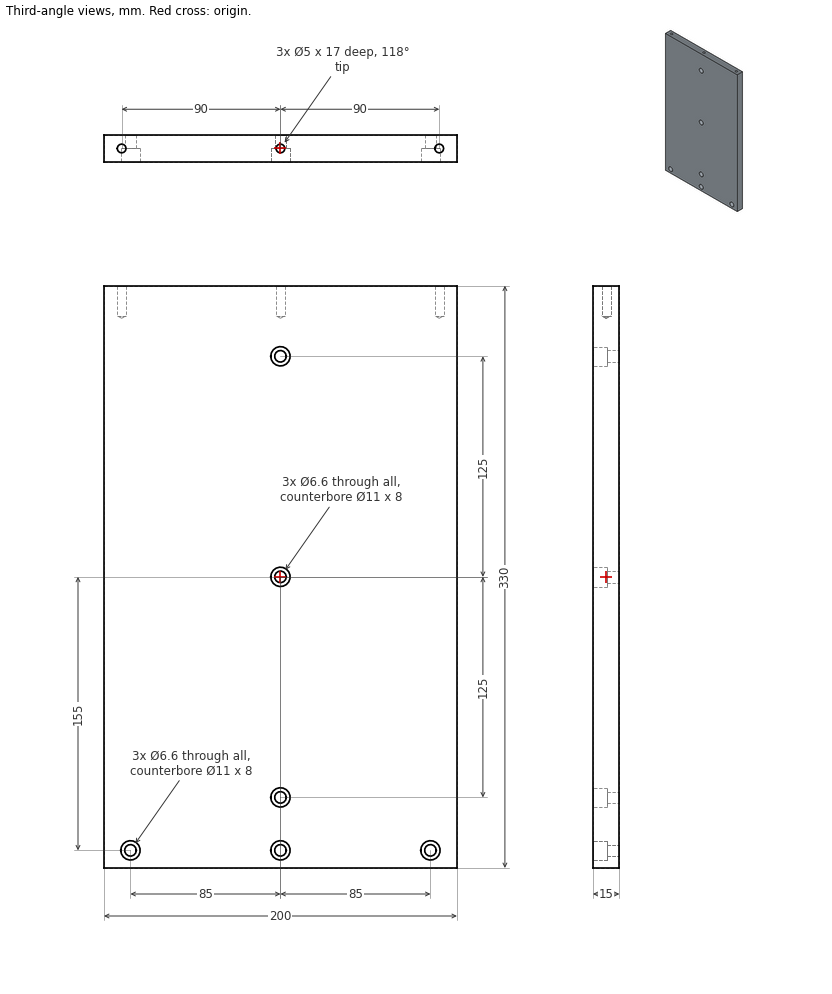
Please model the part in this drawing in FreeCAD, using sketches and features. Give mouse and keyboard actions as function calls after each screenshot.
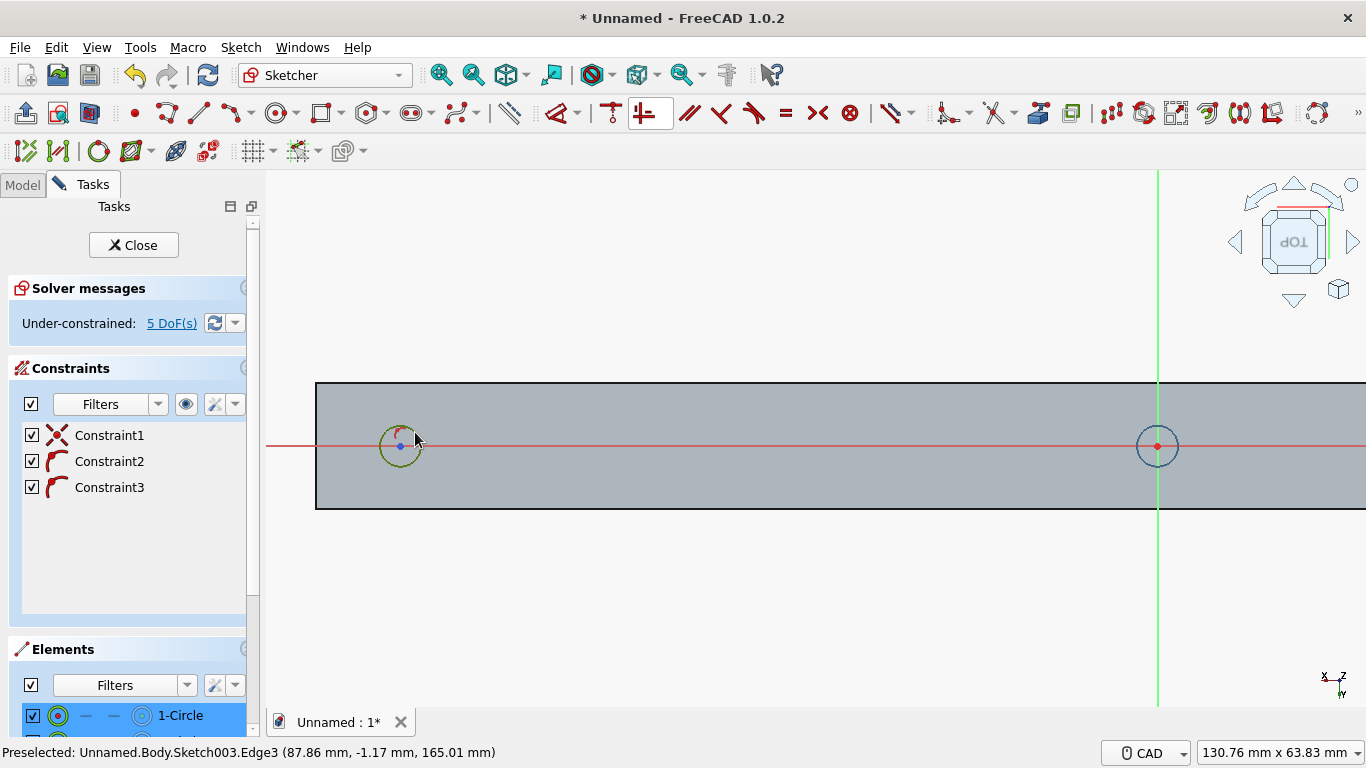
click(786, 114)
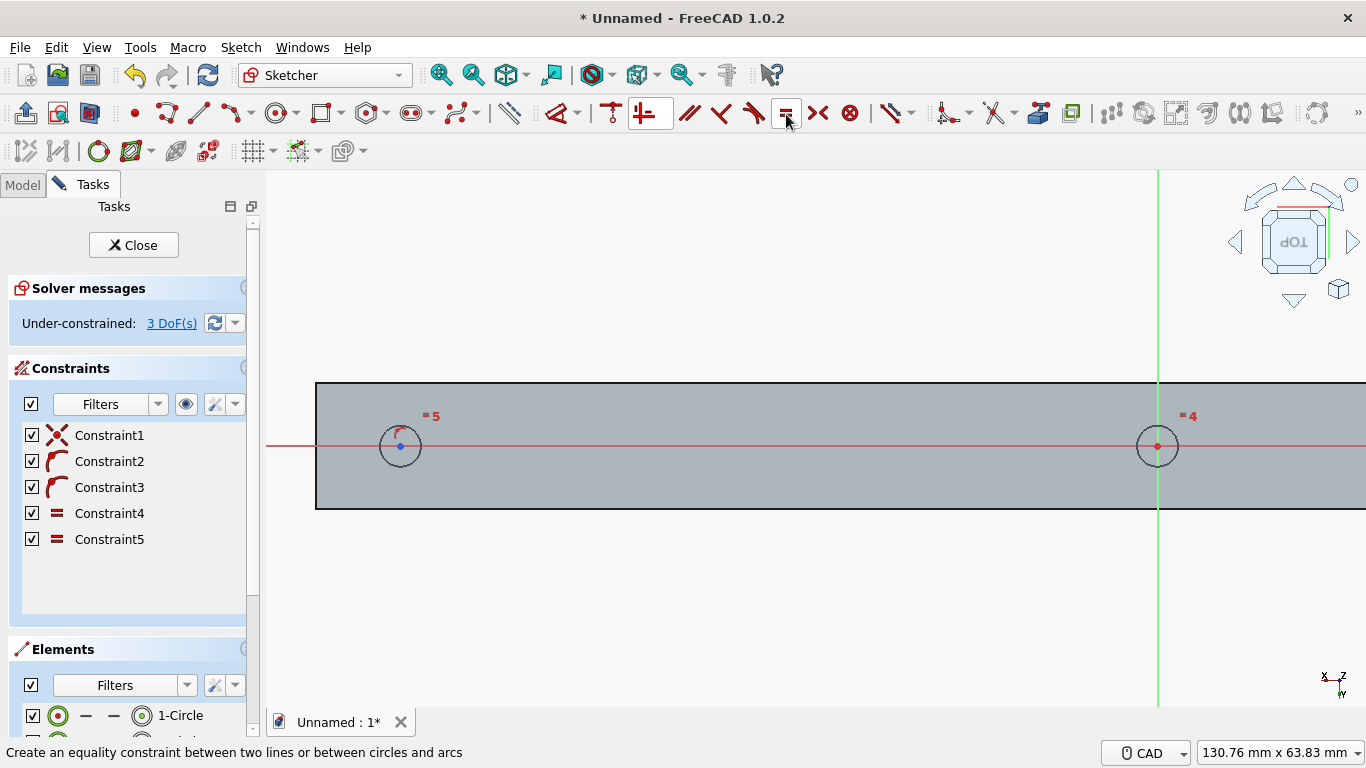
key(d)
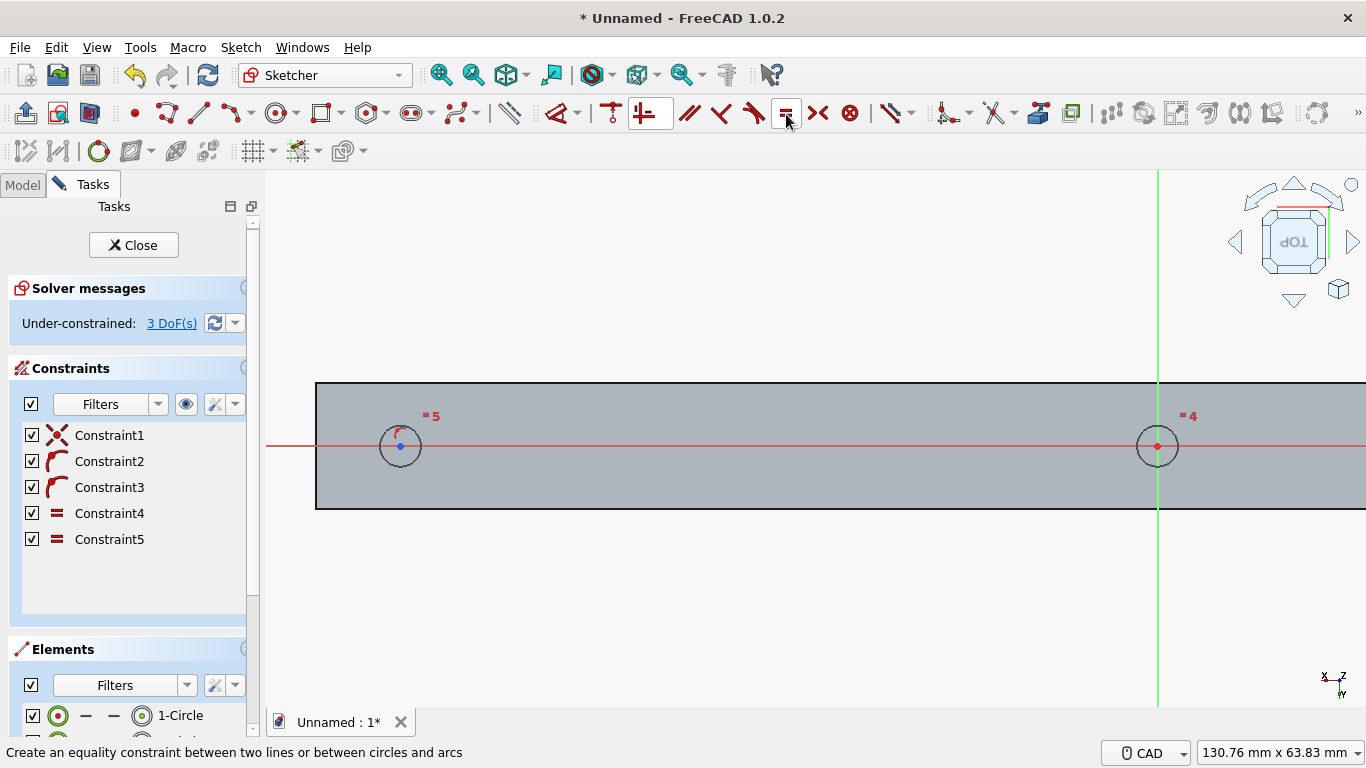
click(1172, 432)
click(1195, 410)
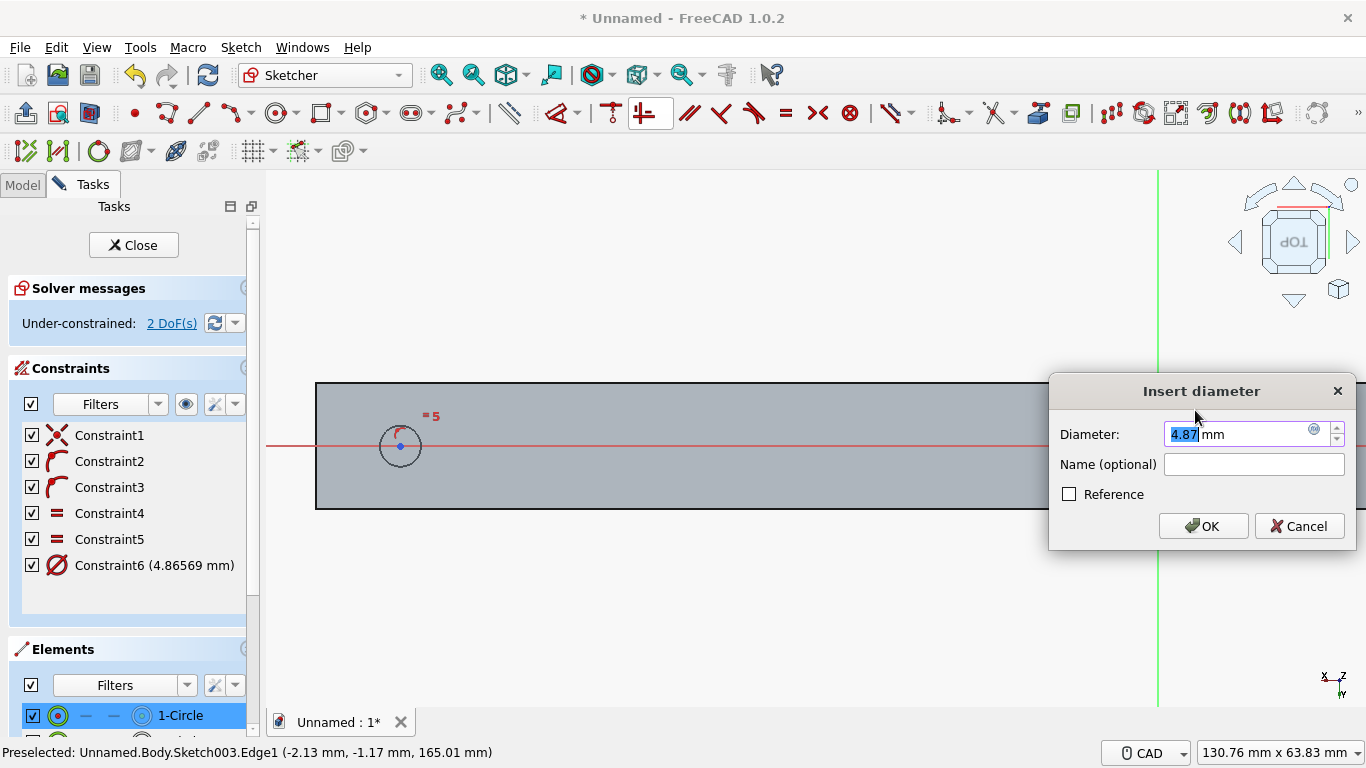
text(5)
key(Return)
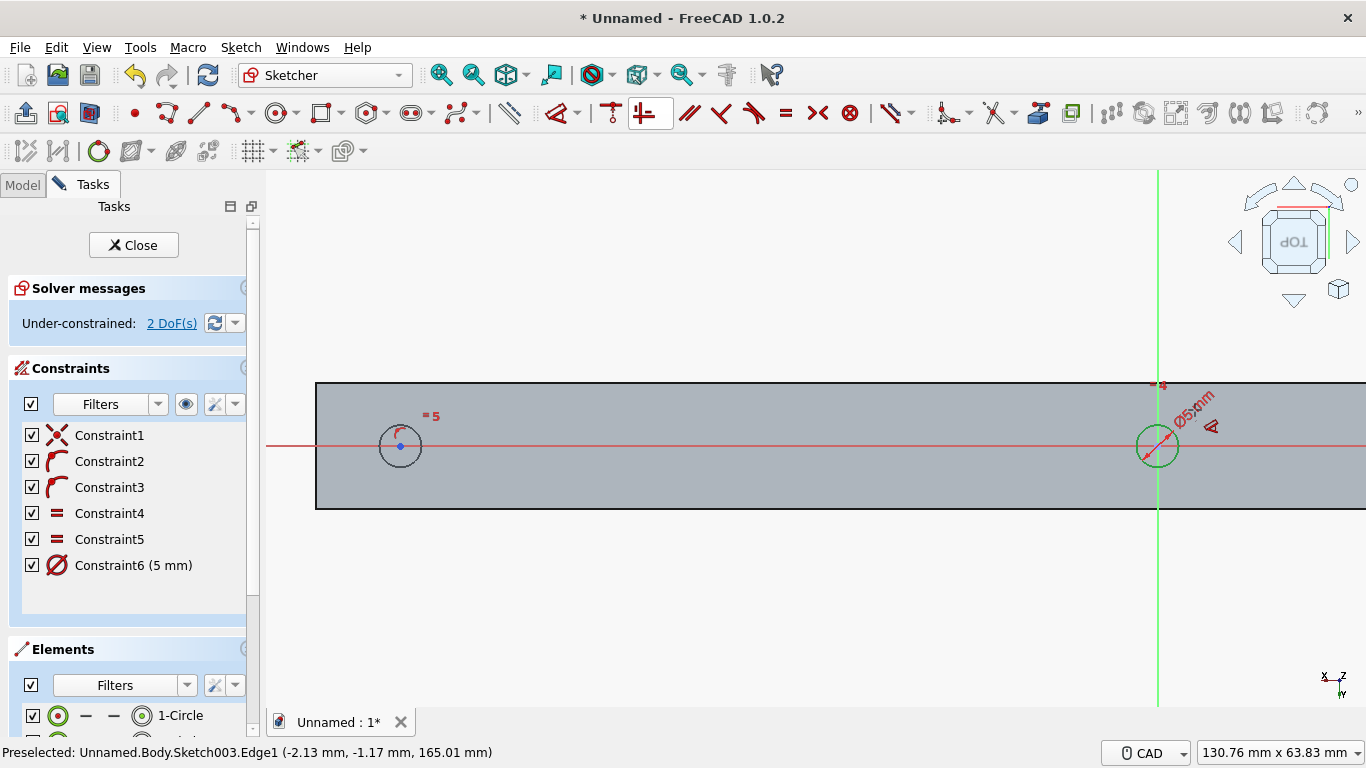
scroll(413, 432, down, 4)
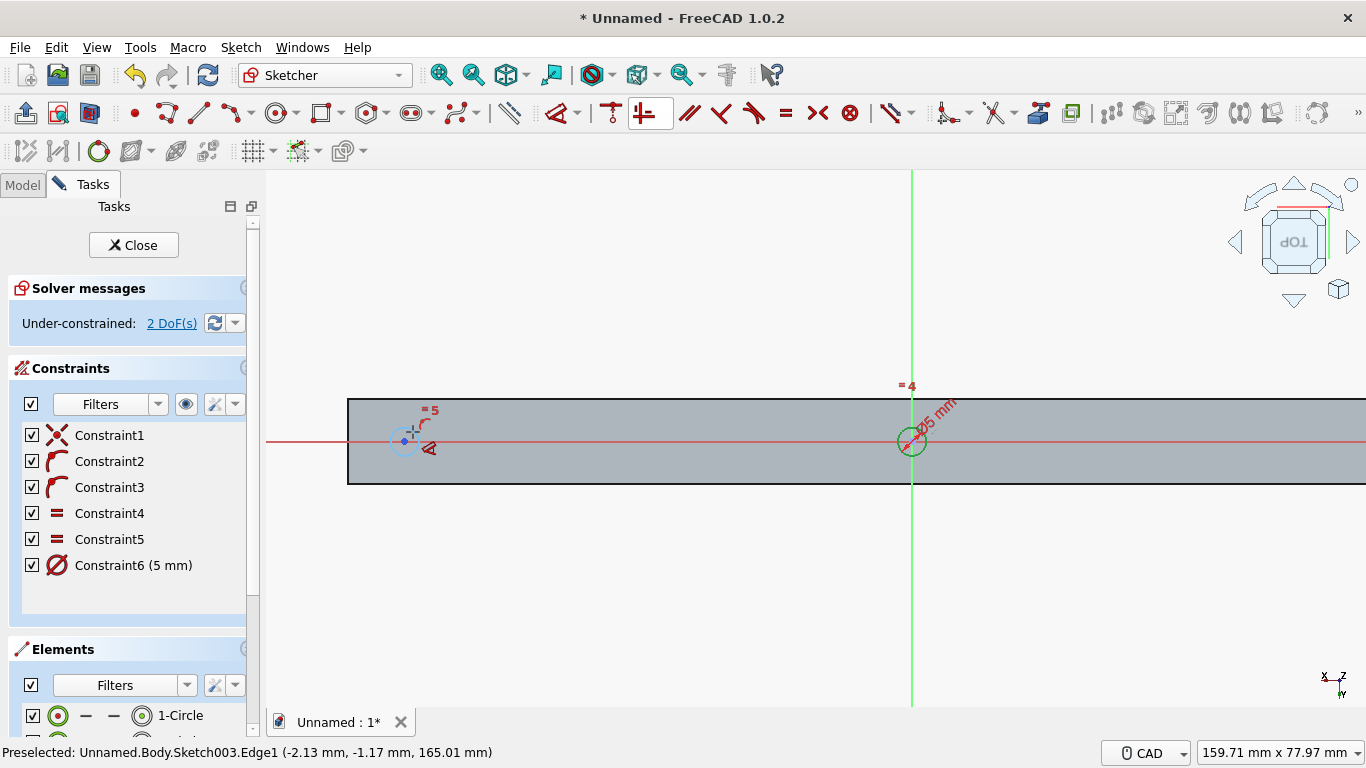
click(1088, 439)
click(918, 473)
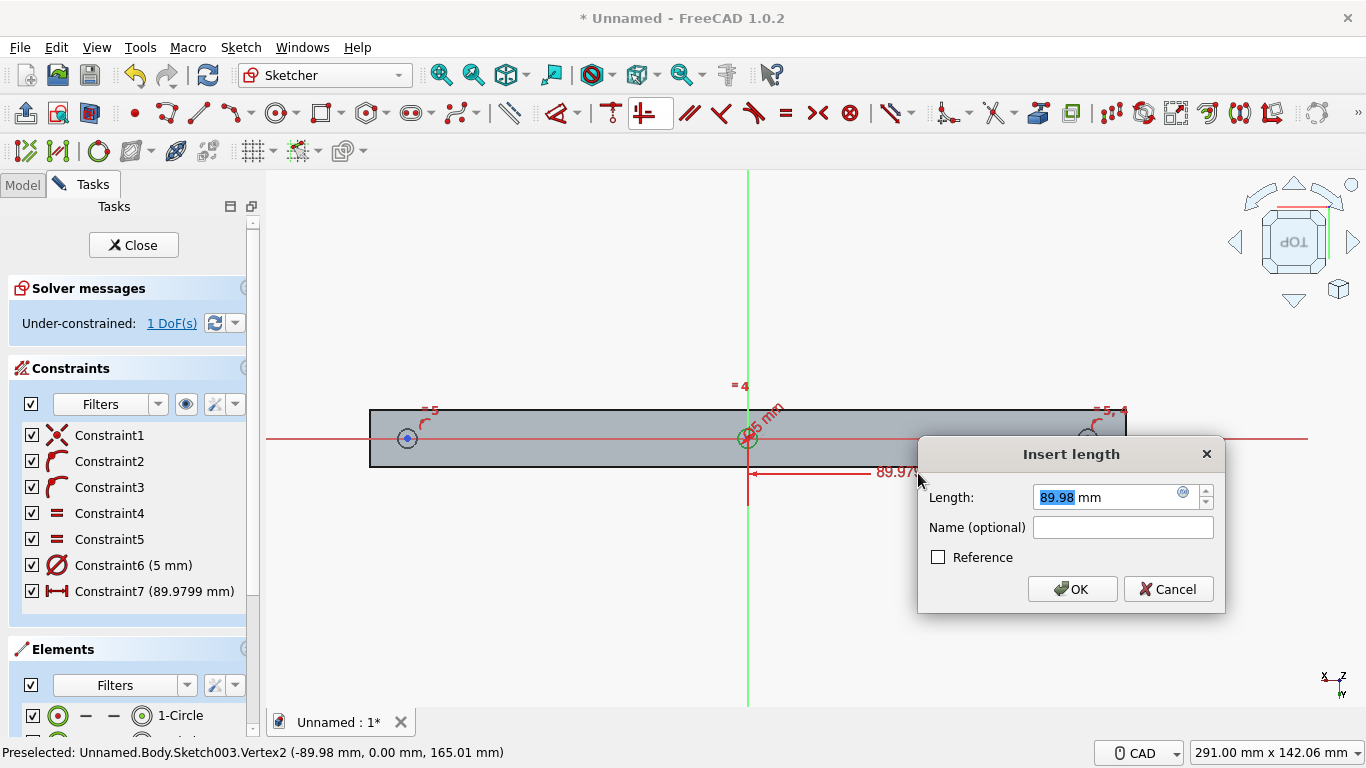
text(90)
key(Return)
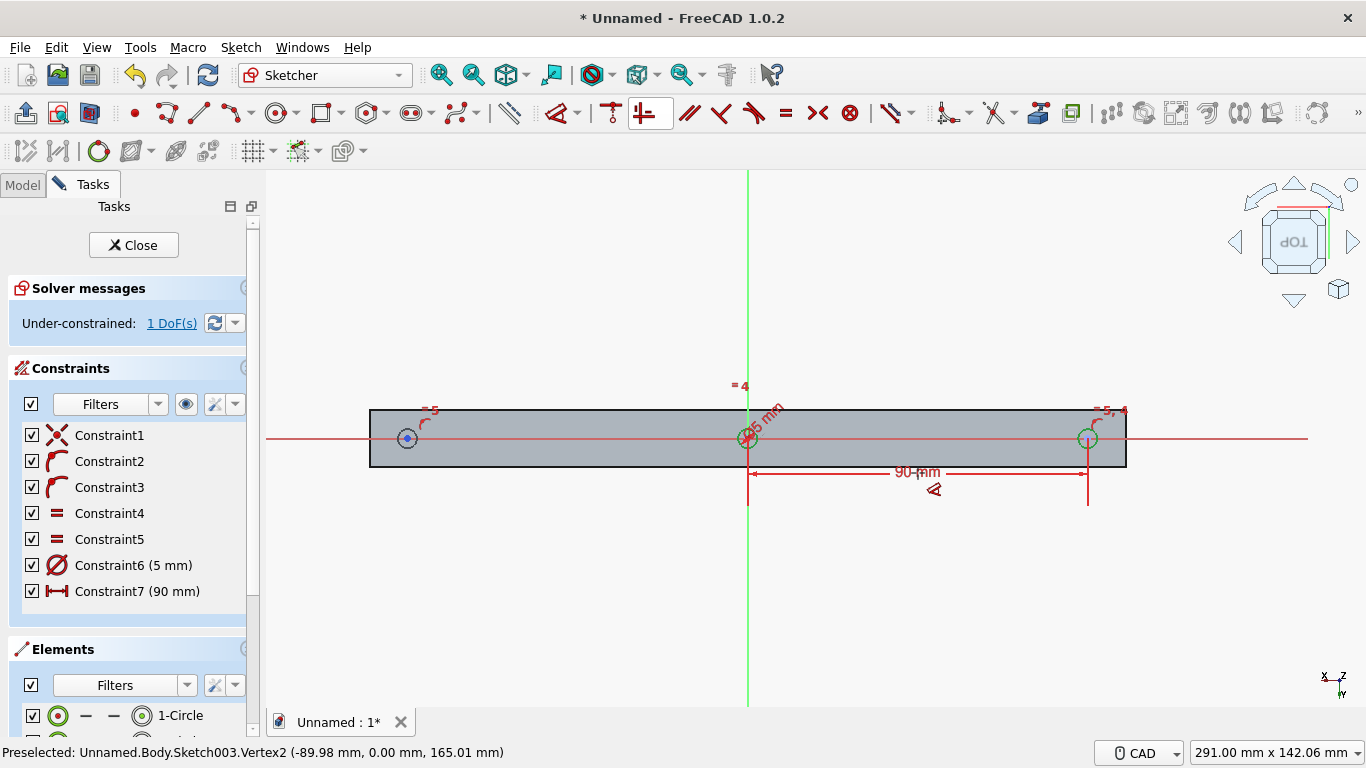
click(407, 439)
click(578, 473)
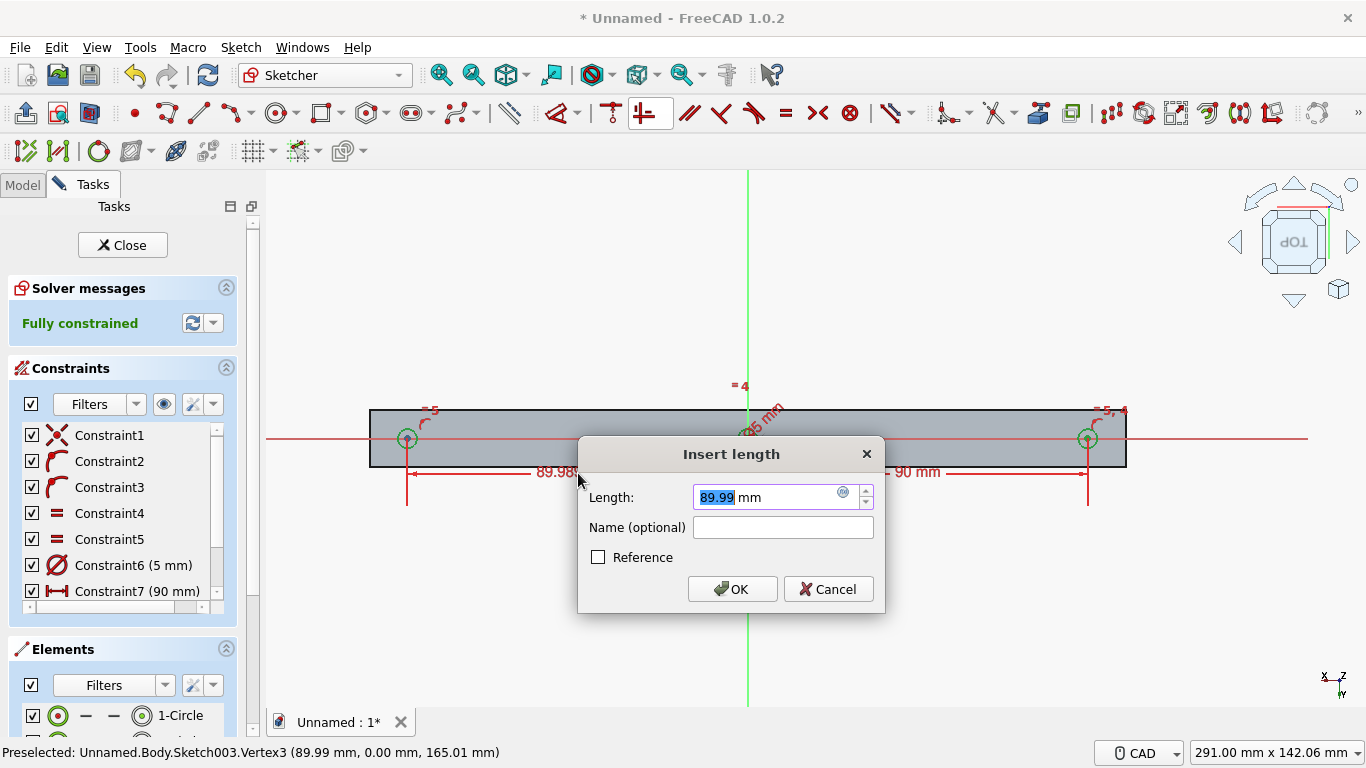
text(90)
key(Return)
key(Escape)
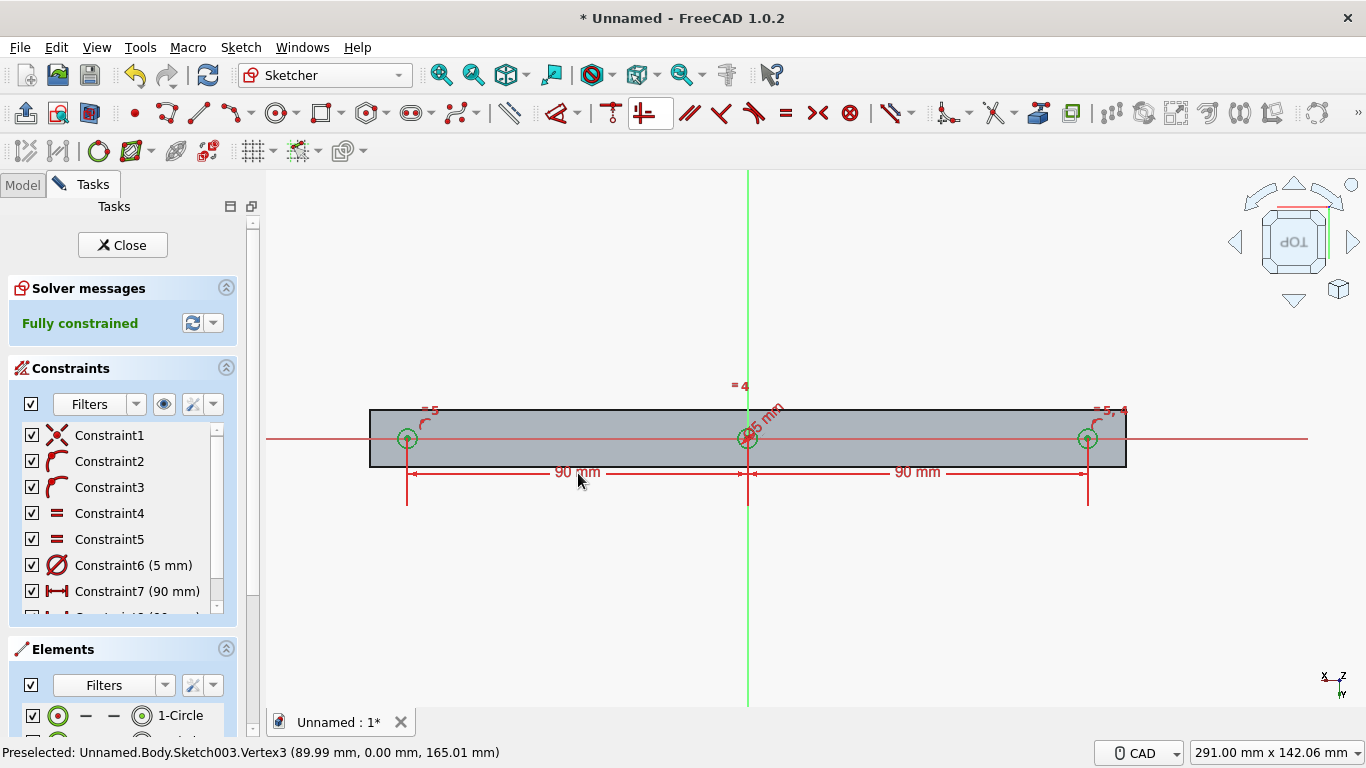
click(123, 245)